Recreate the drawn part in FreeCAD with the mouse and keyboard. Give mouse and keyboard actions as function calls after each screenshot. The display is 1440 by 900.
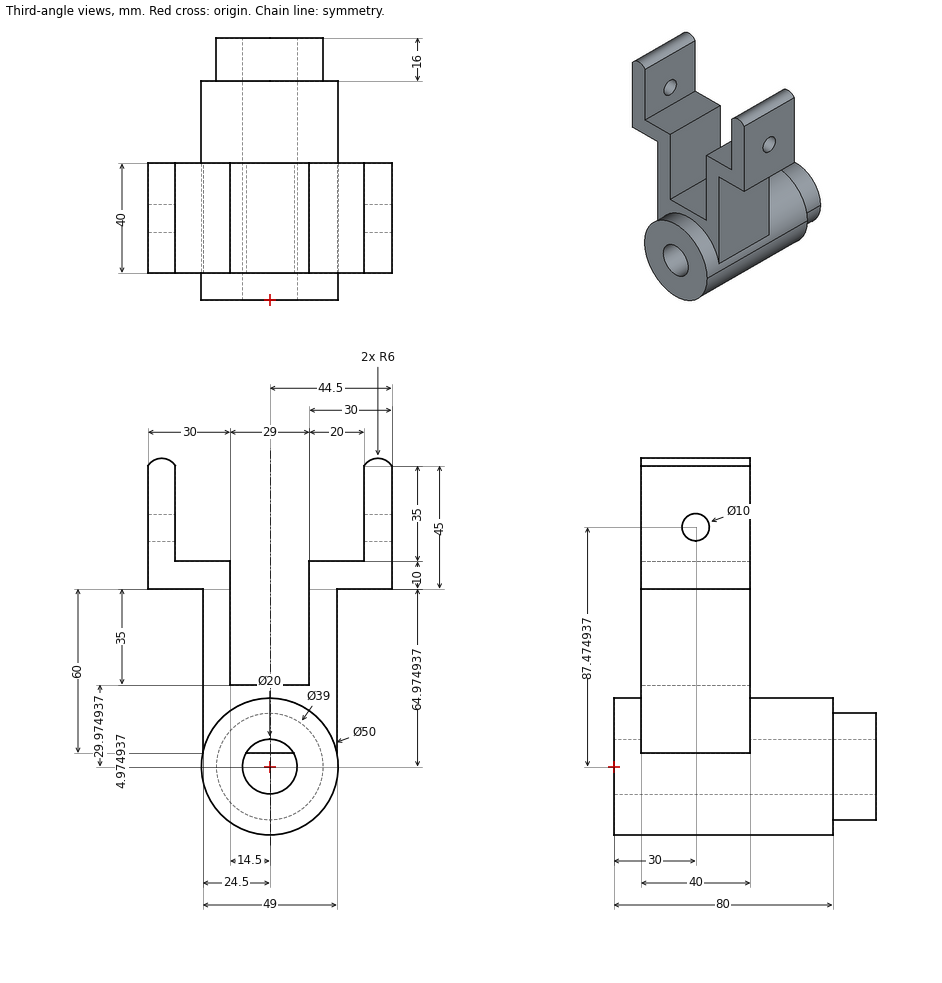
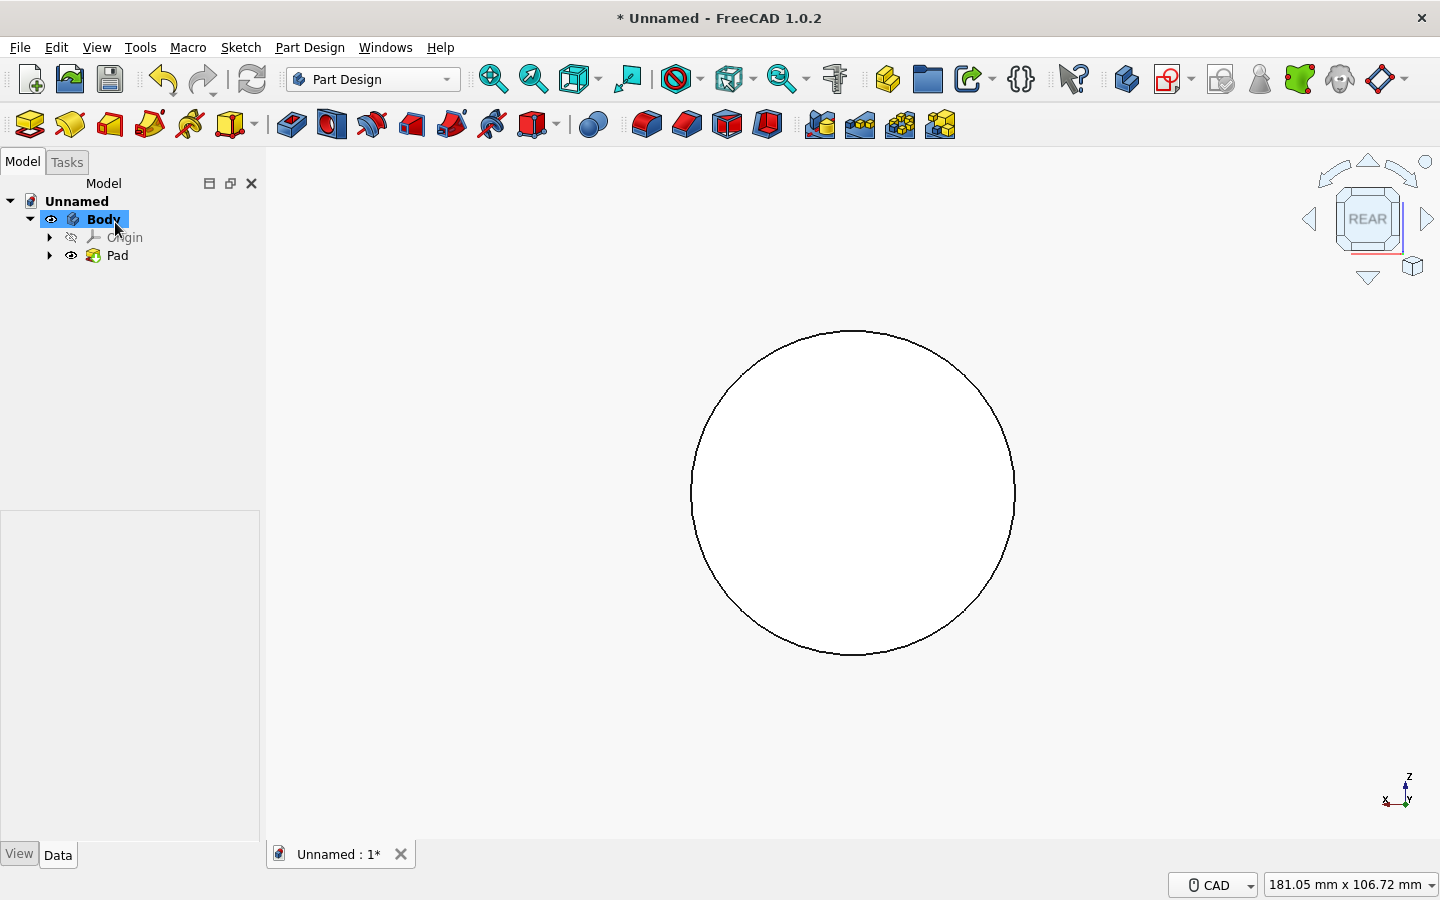
click(853, 492)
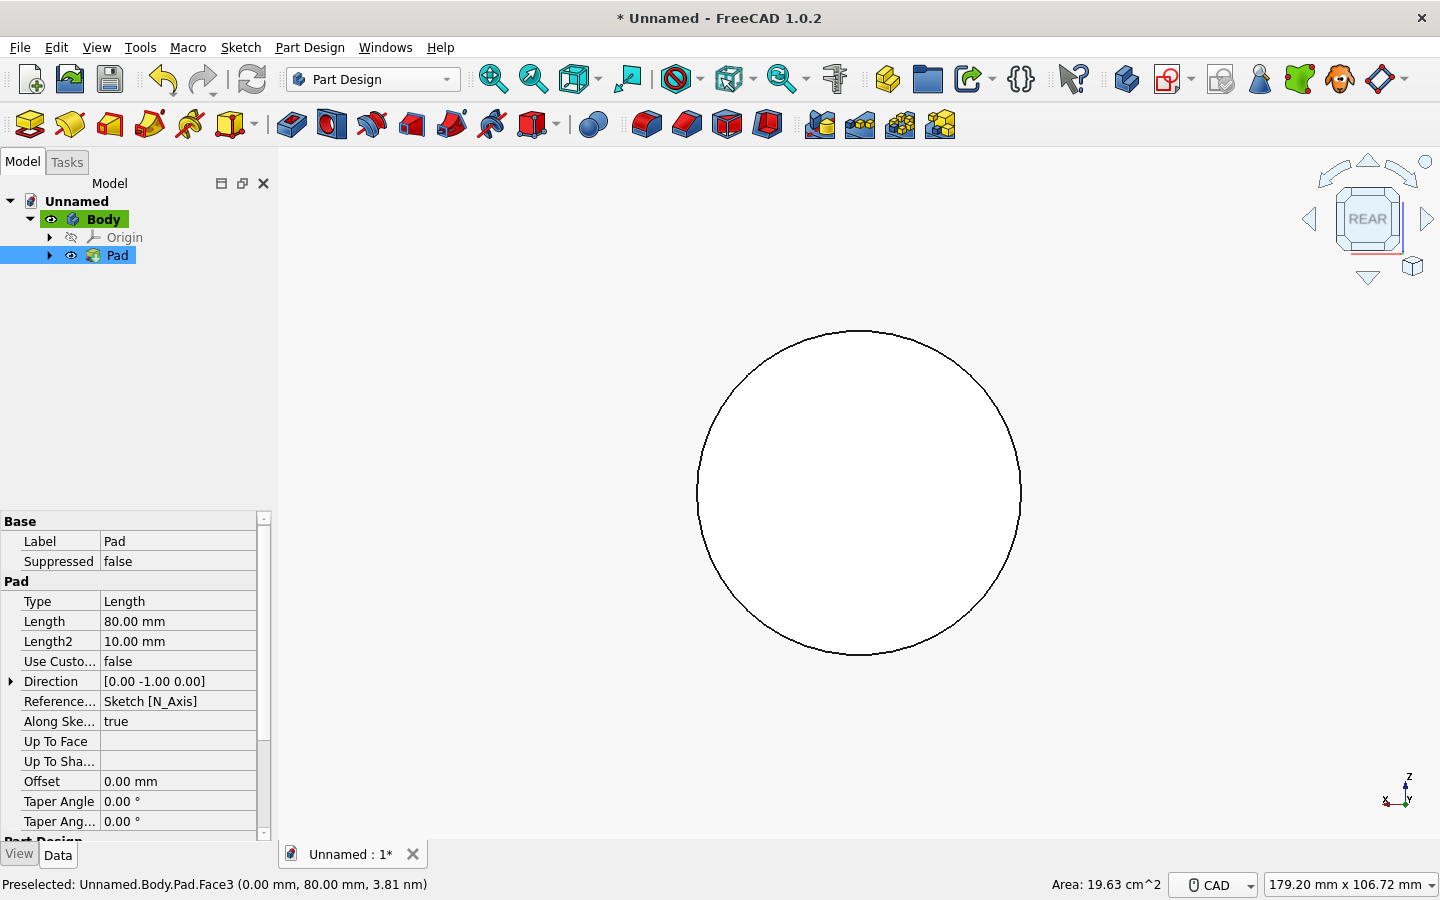
click(1168, 80)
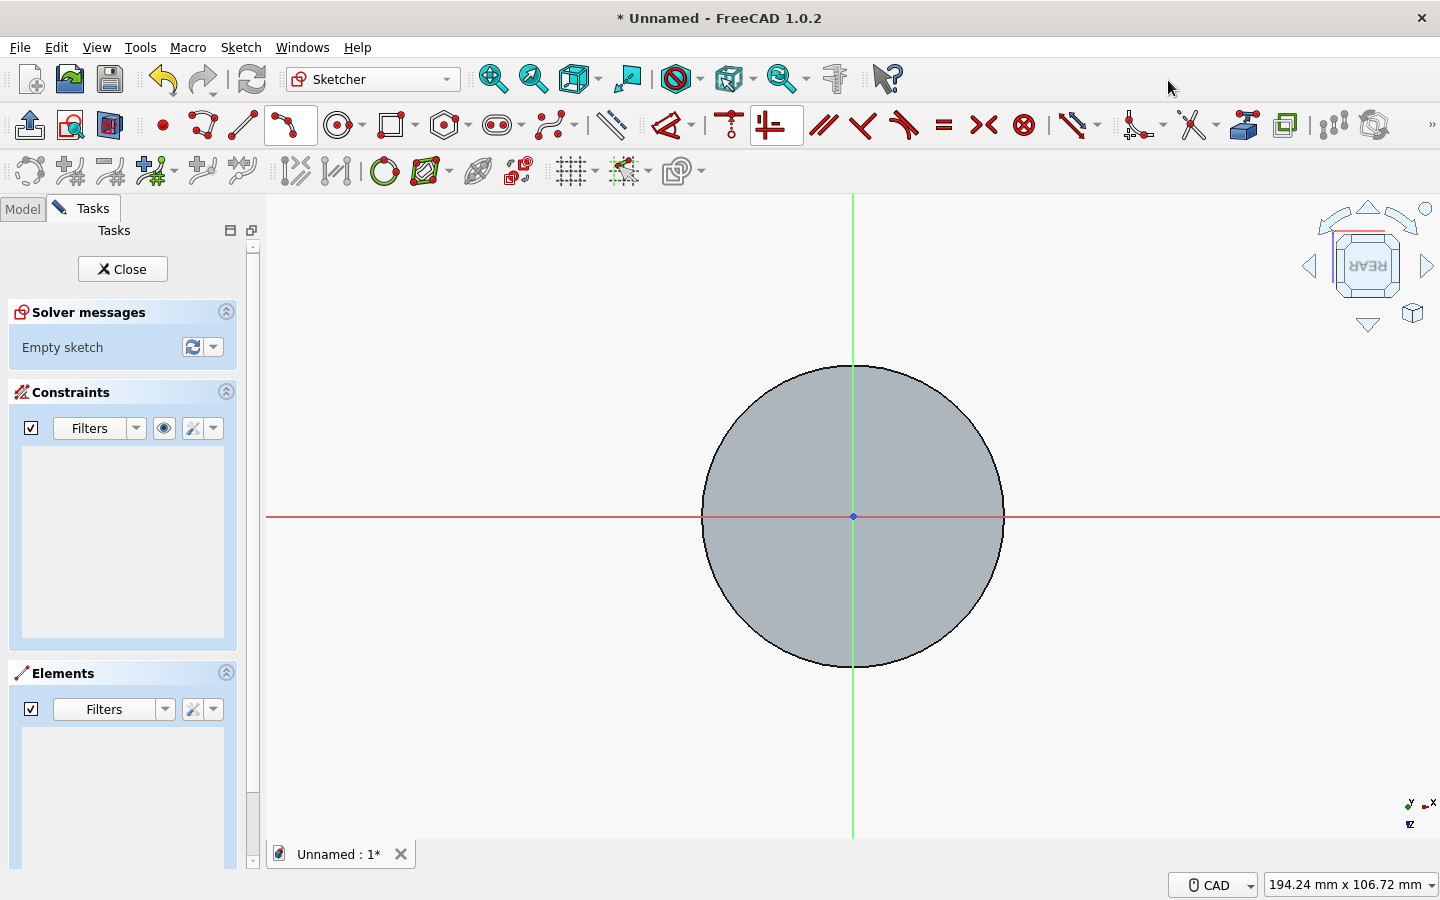
scroll(936, 516, up, 3)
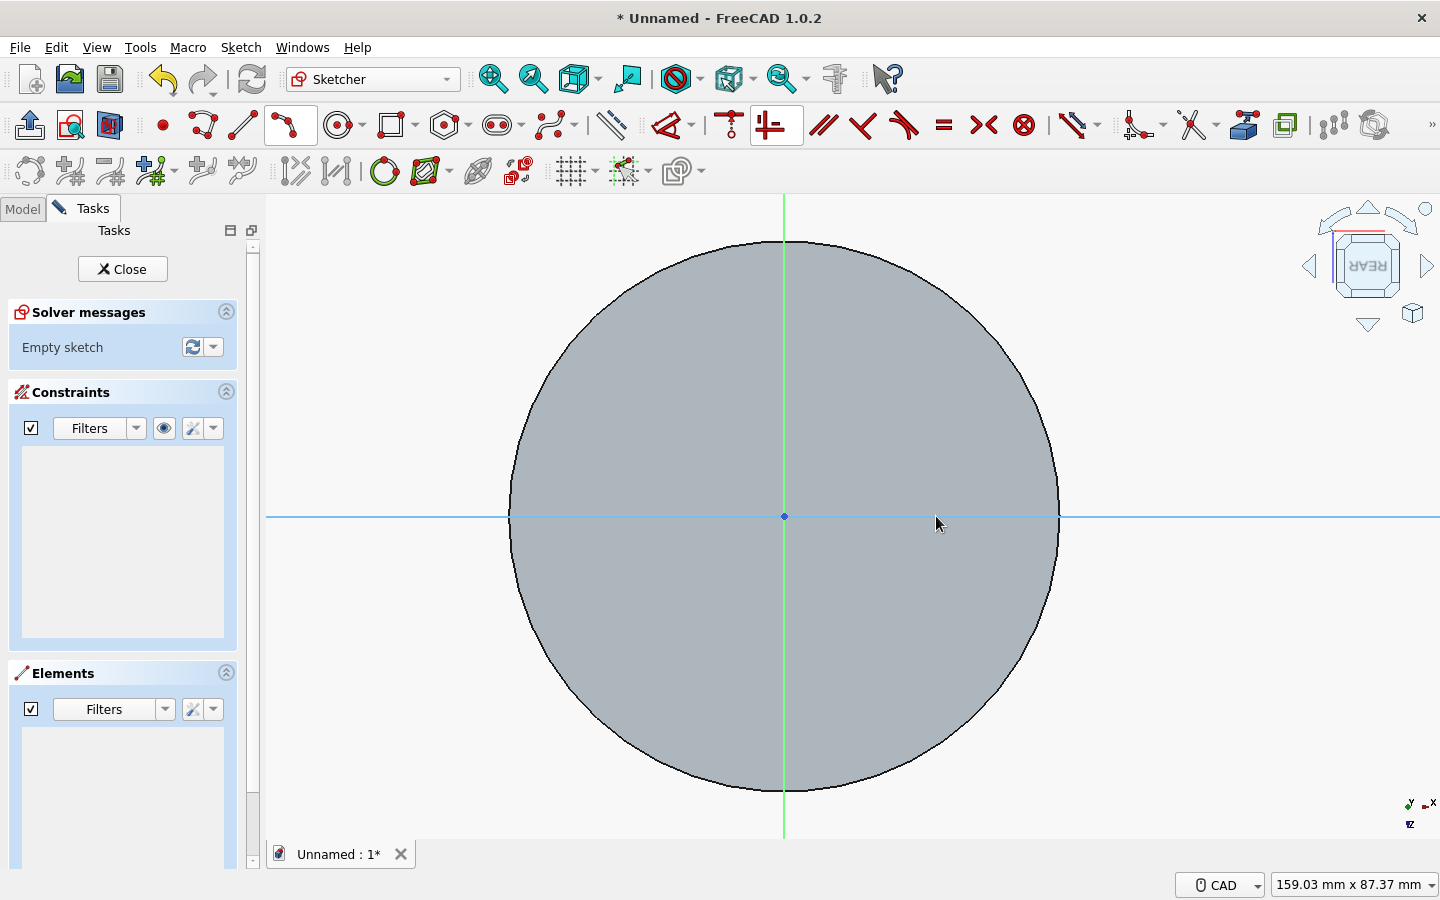
click(338, 126)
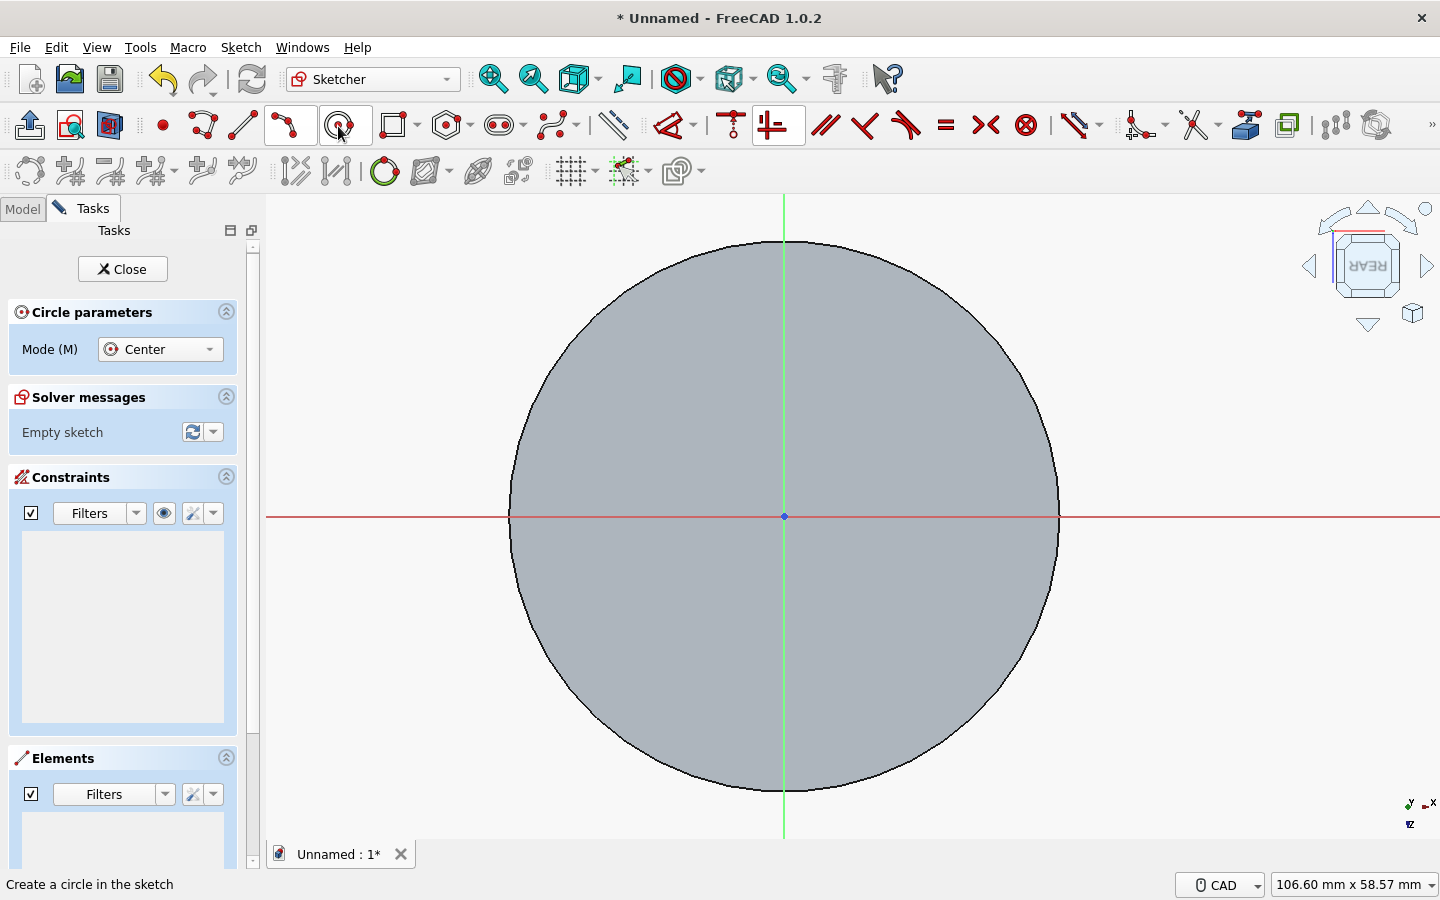
click(784, 516)
click(936, 365)
key(Escape)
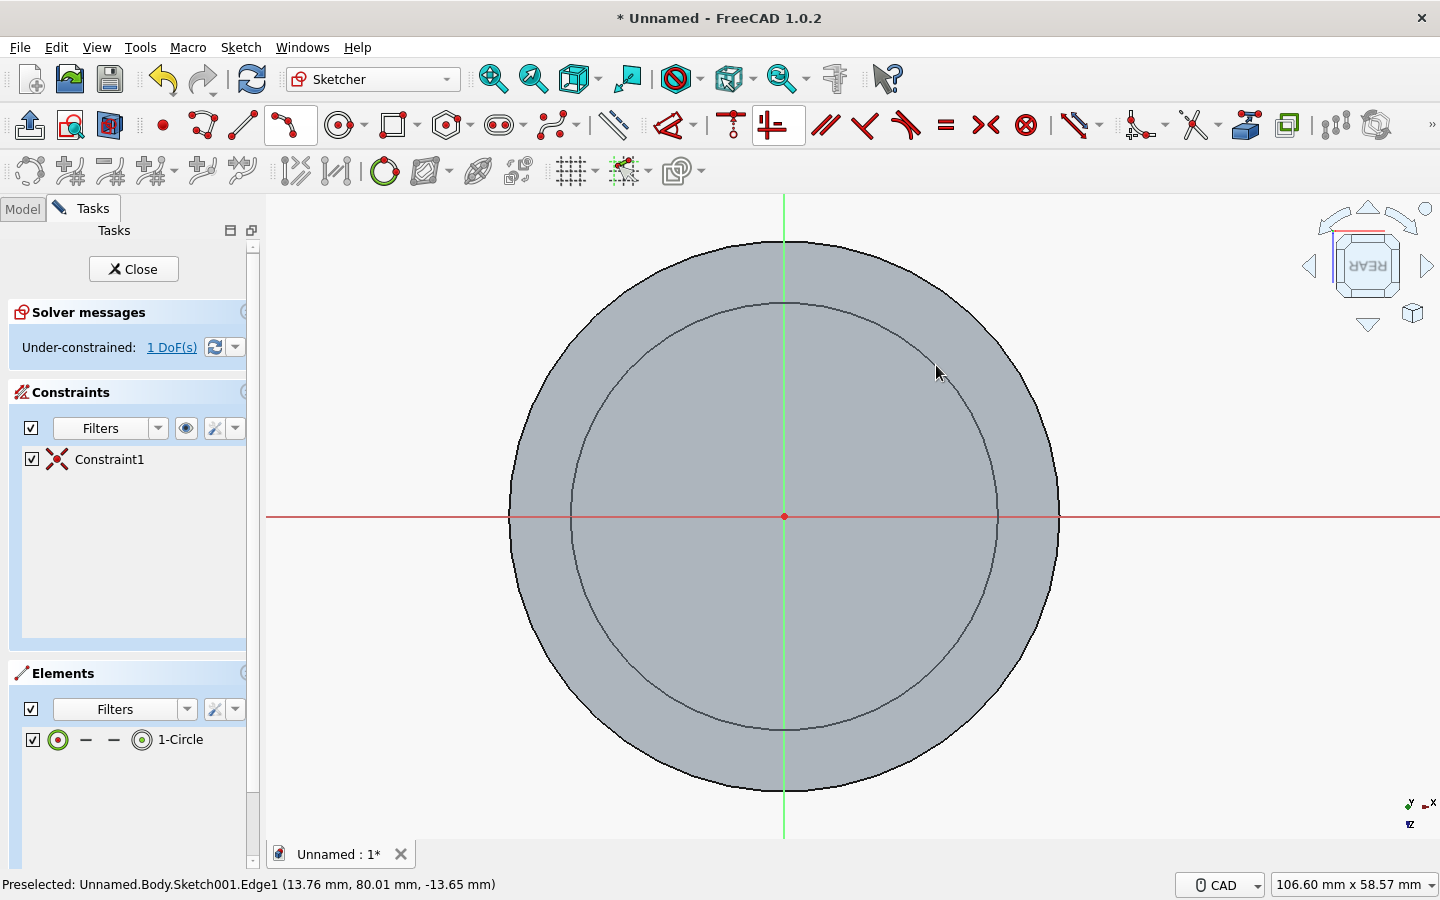
click(668, 126)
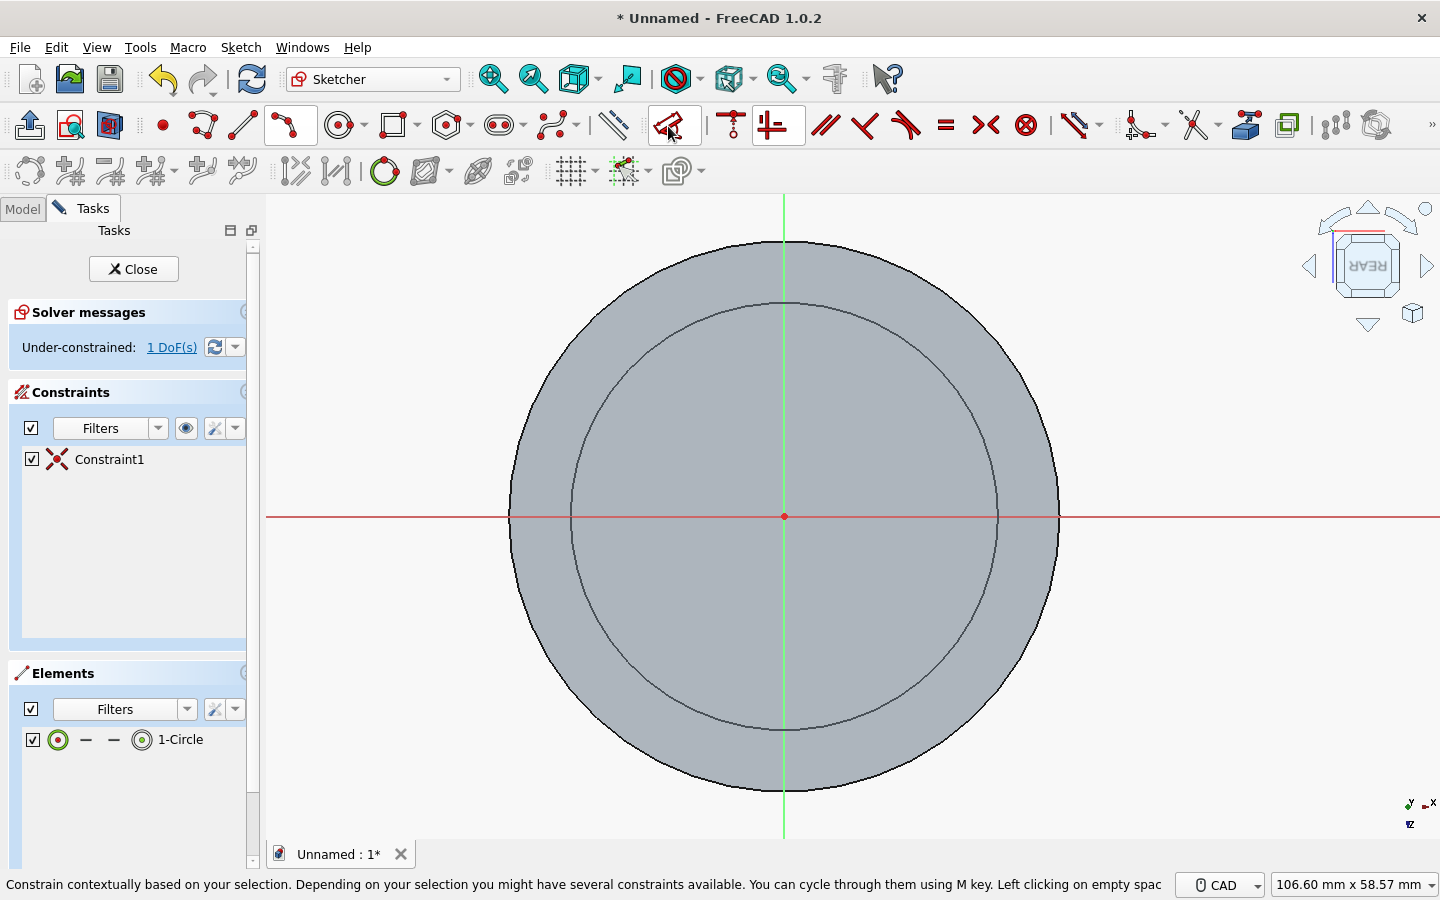
click(935, 365)
click(958, 342)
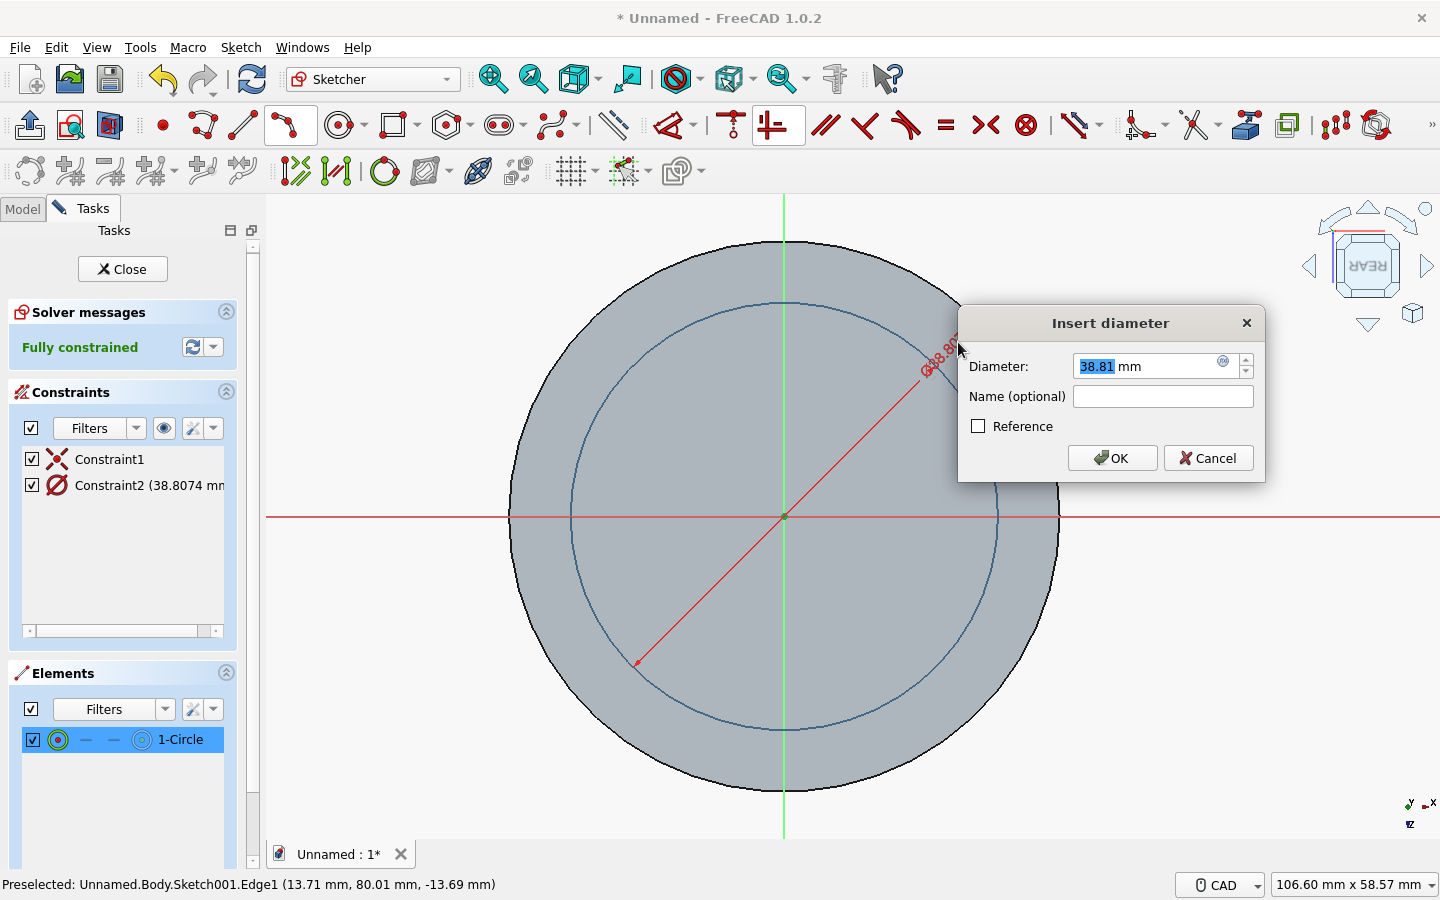
text(39)
key(Return)
key(Escape)